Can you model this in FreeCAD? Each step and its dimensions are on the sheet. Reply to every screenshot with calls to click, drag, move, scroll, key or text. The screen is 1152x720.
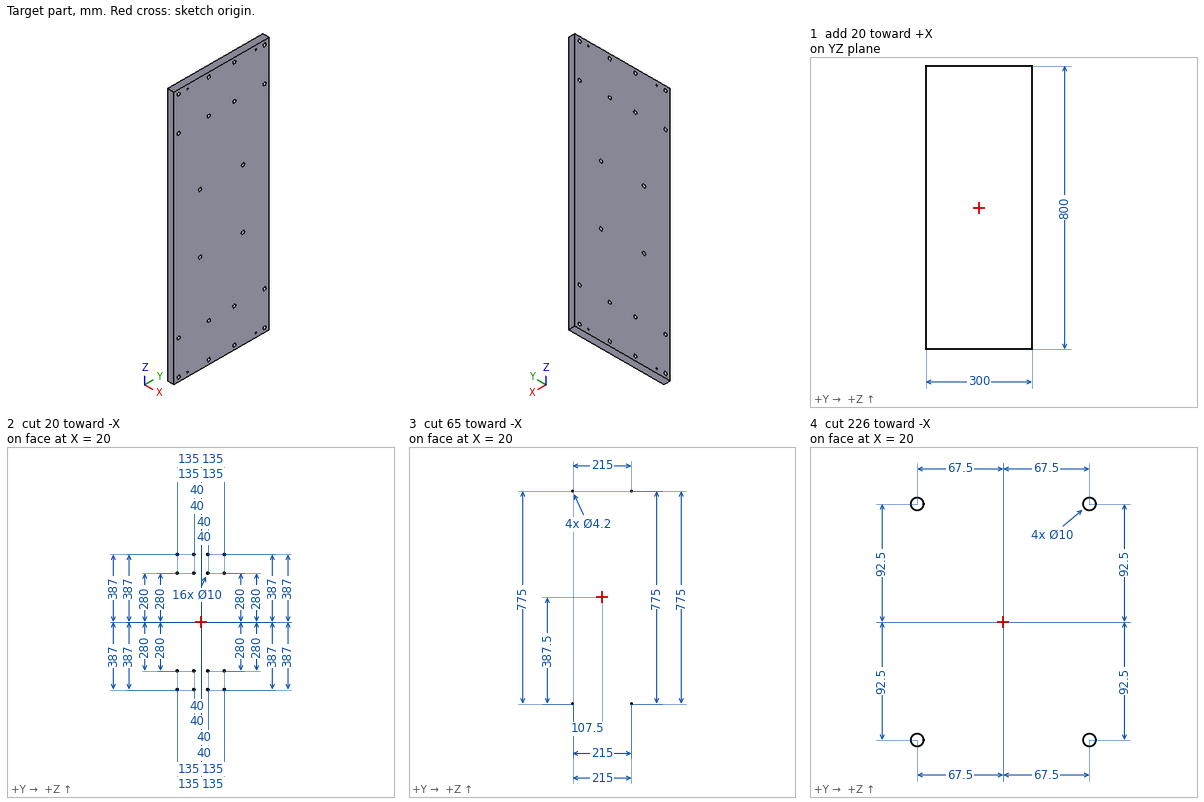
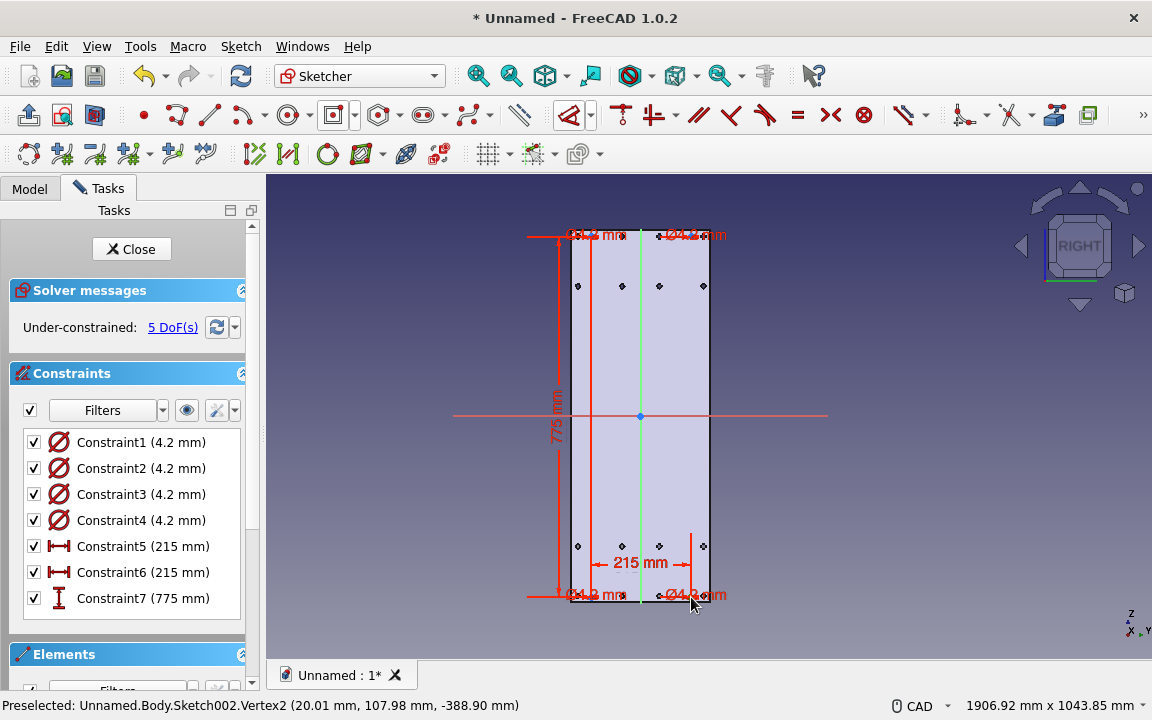
click(591, 237)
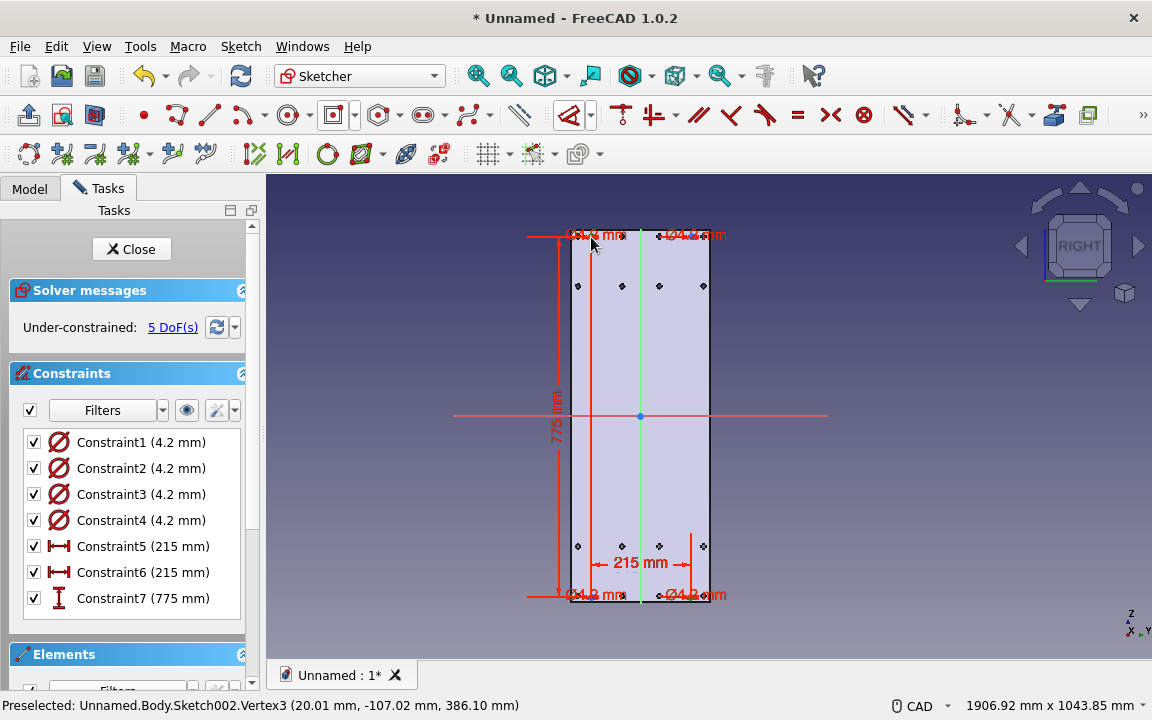
key(i)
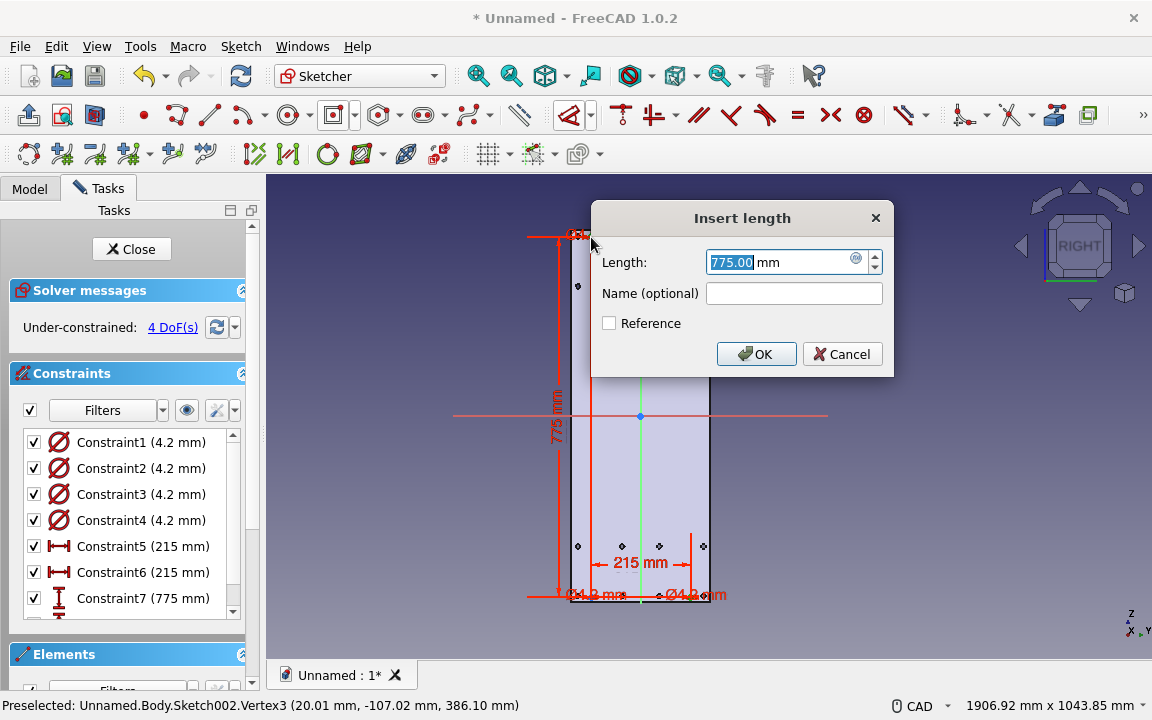
text(775)
key(Return)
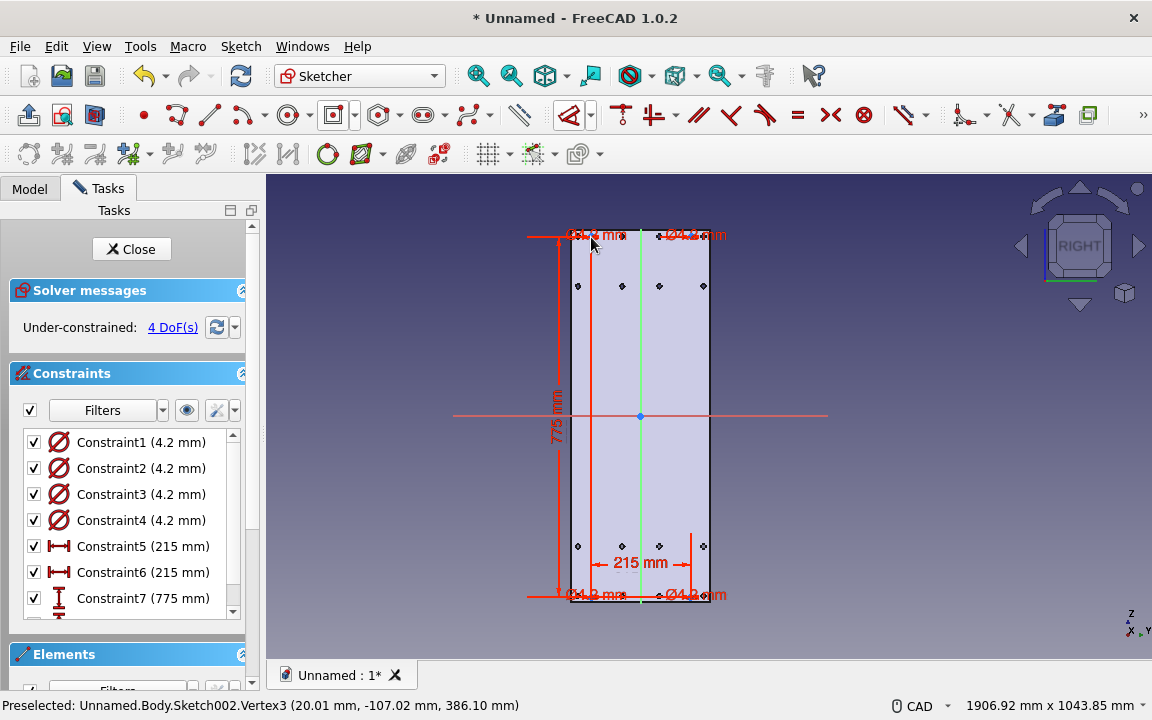
click(591, 237)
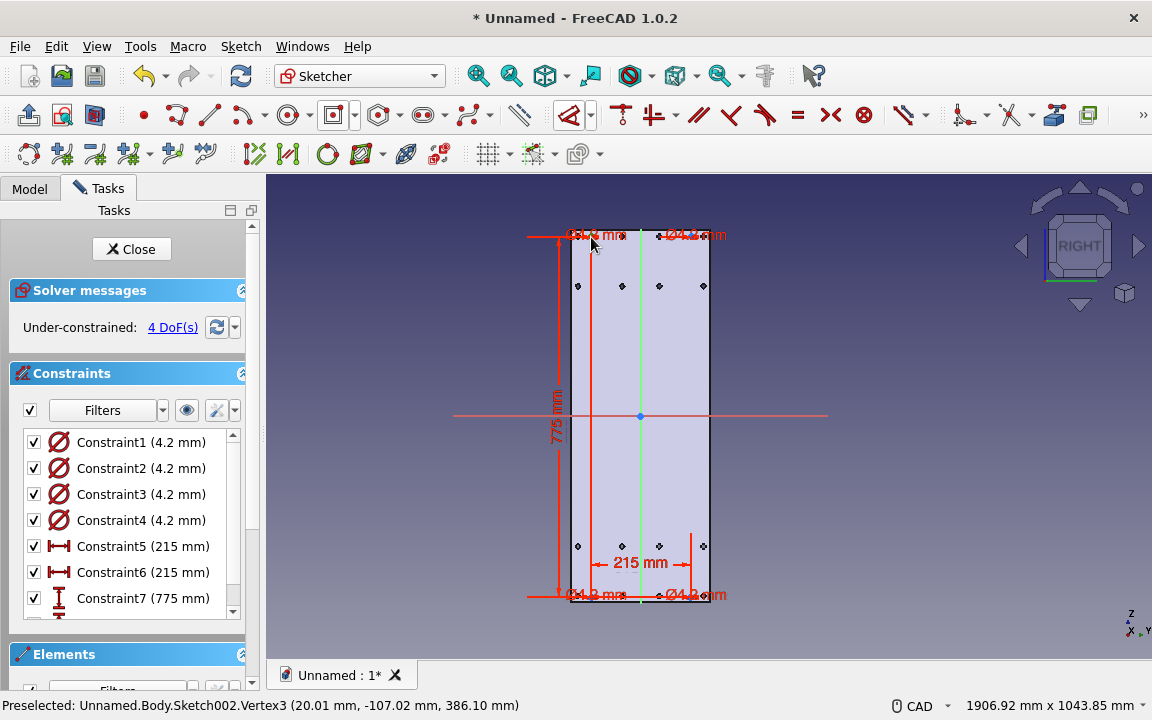
click(691, 237)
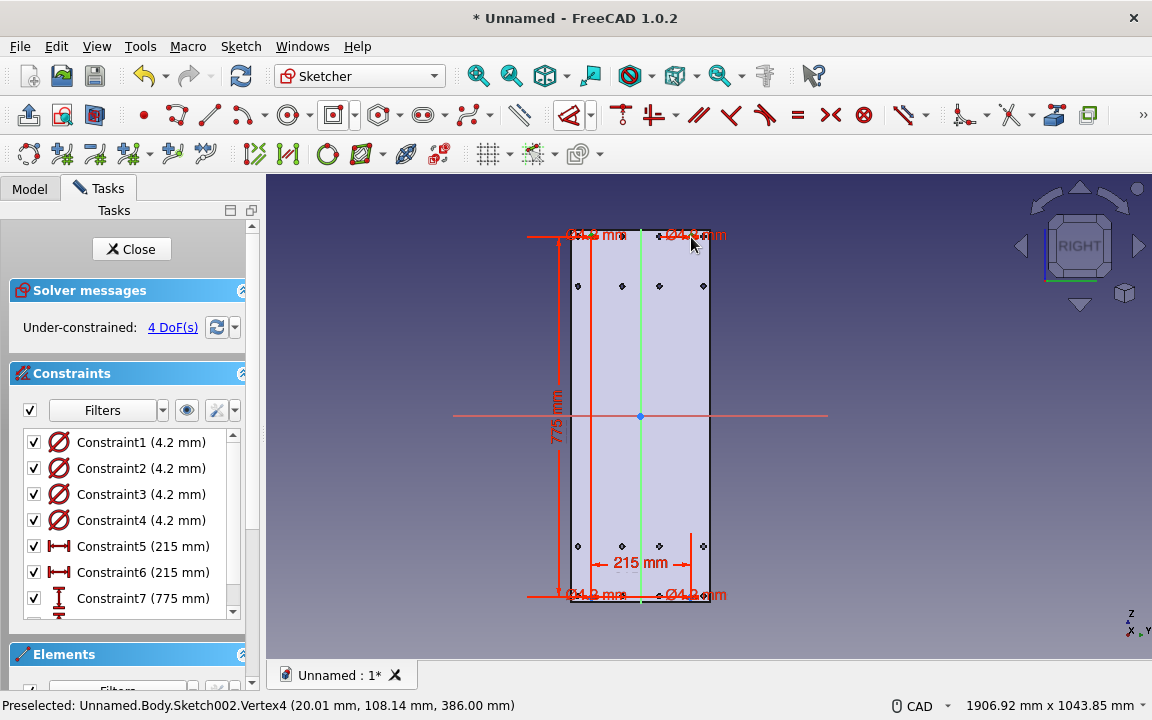
click(590, 116)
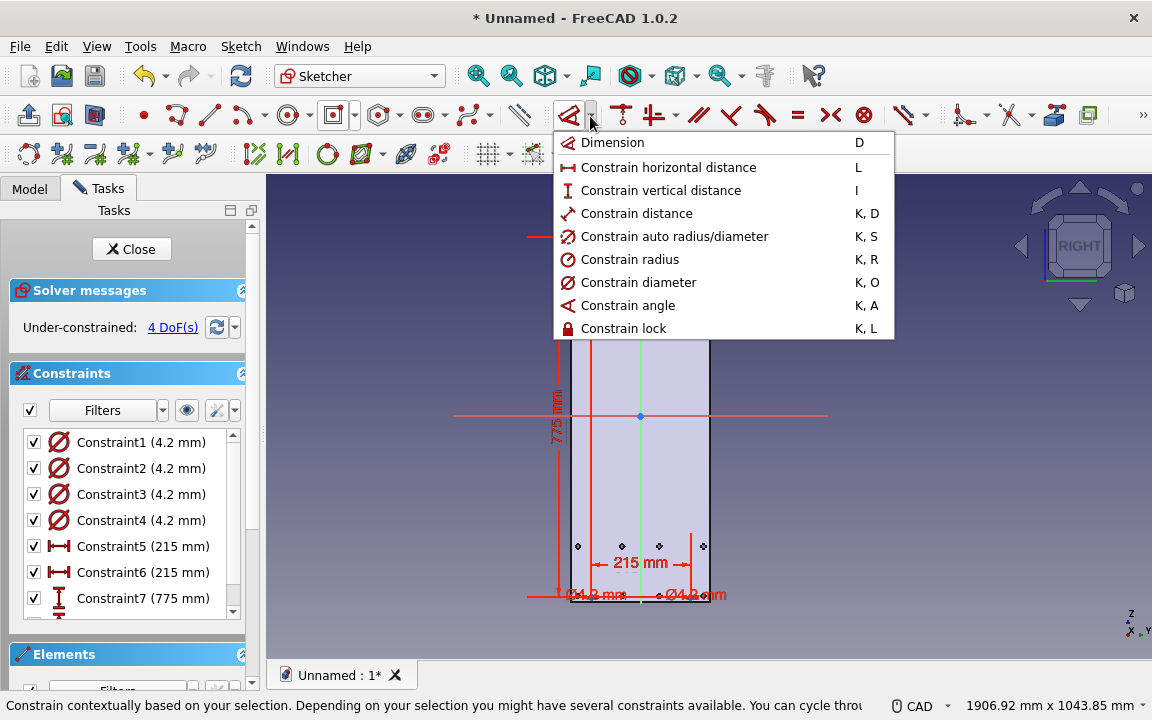
click(724, 168)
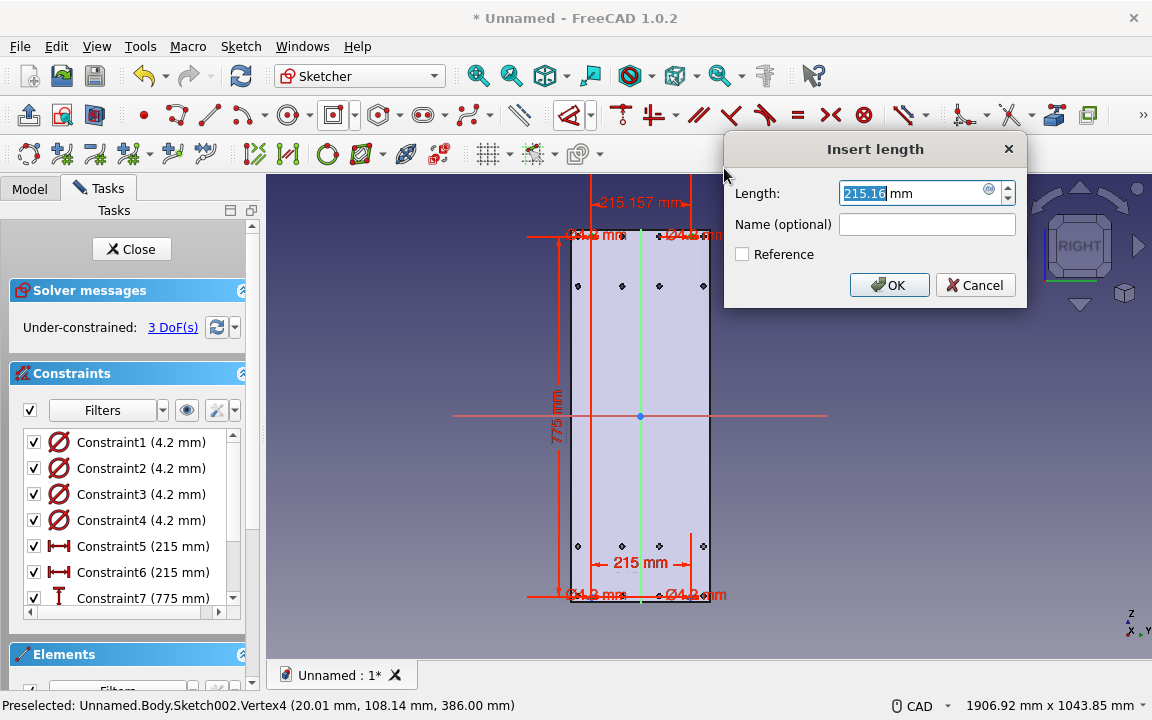
text(215)
key(Return)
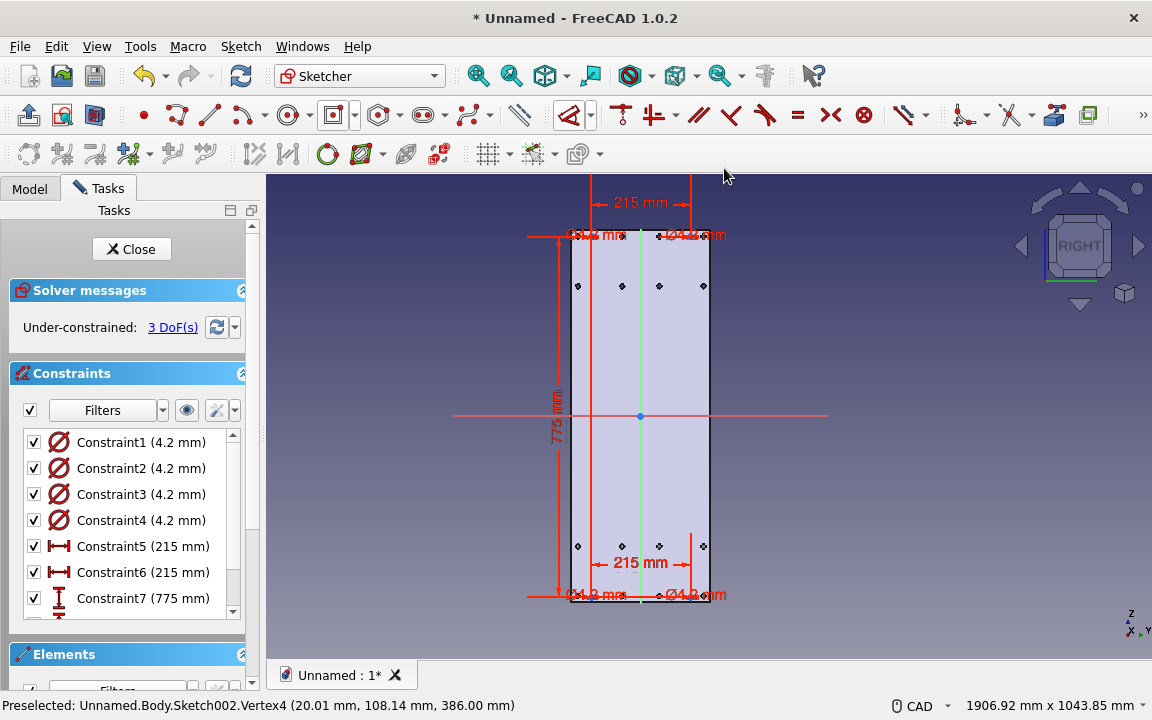
click(691, 597)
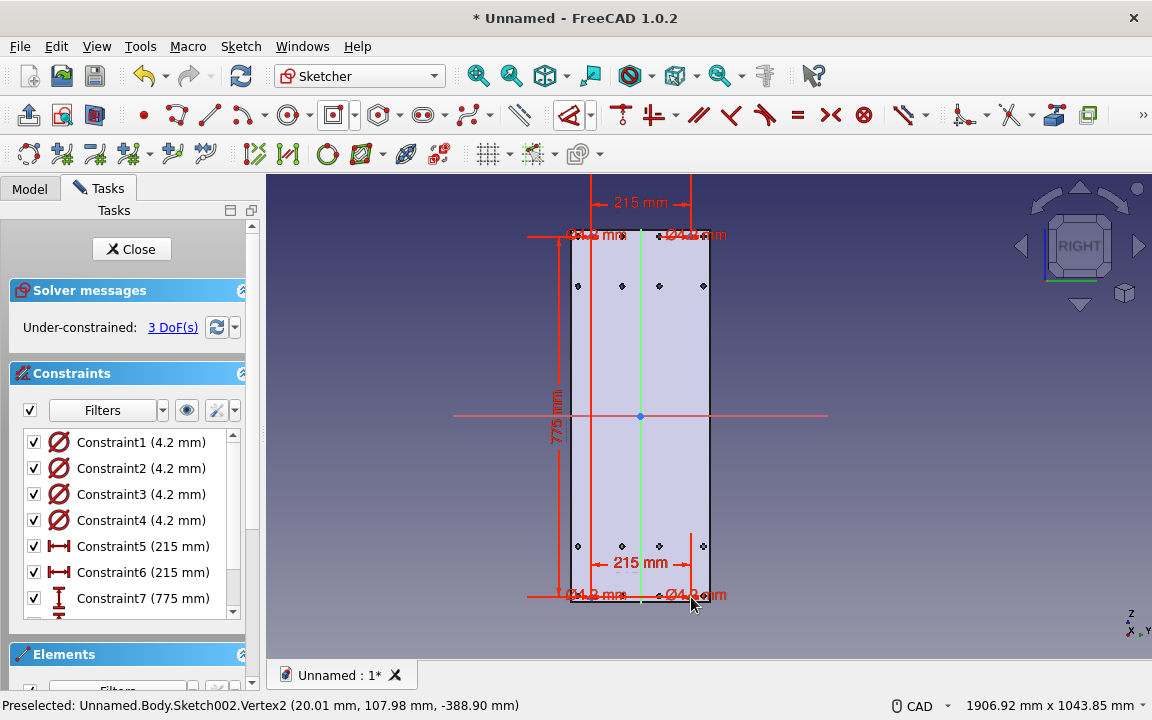
click(691, 237)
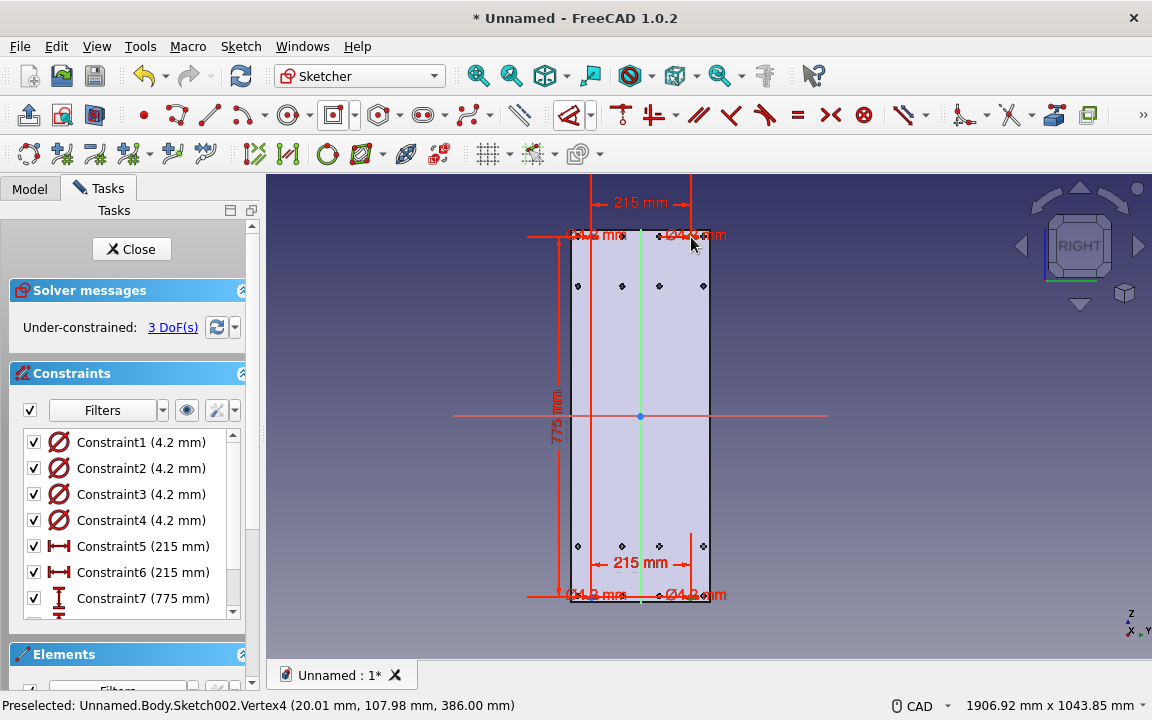
key(i)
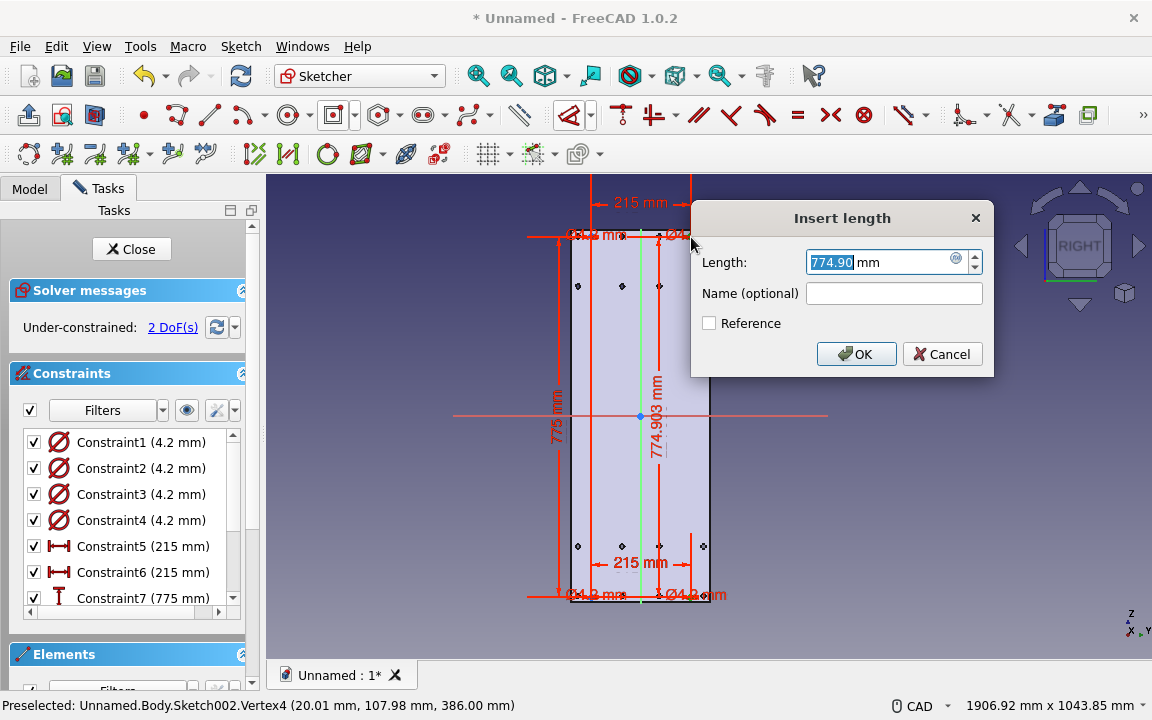
text(775)
key(Return)